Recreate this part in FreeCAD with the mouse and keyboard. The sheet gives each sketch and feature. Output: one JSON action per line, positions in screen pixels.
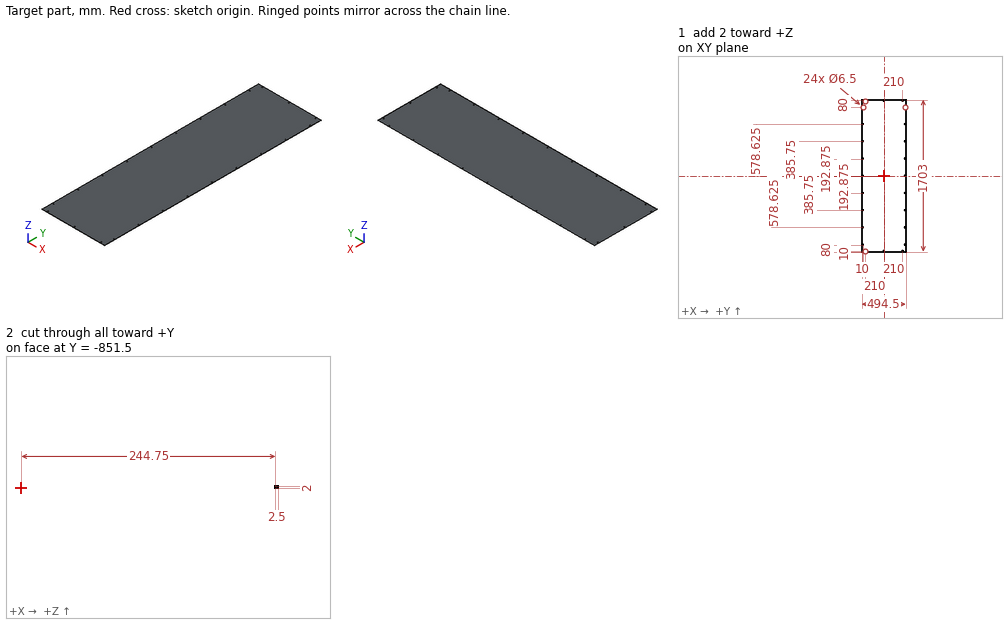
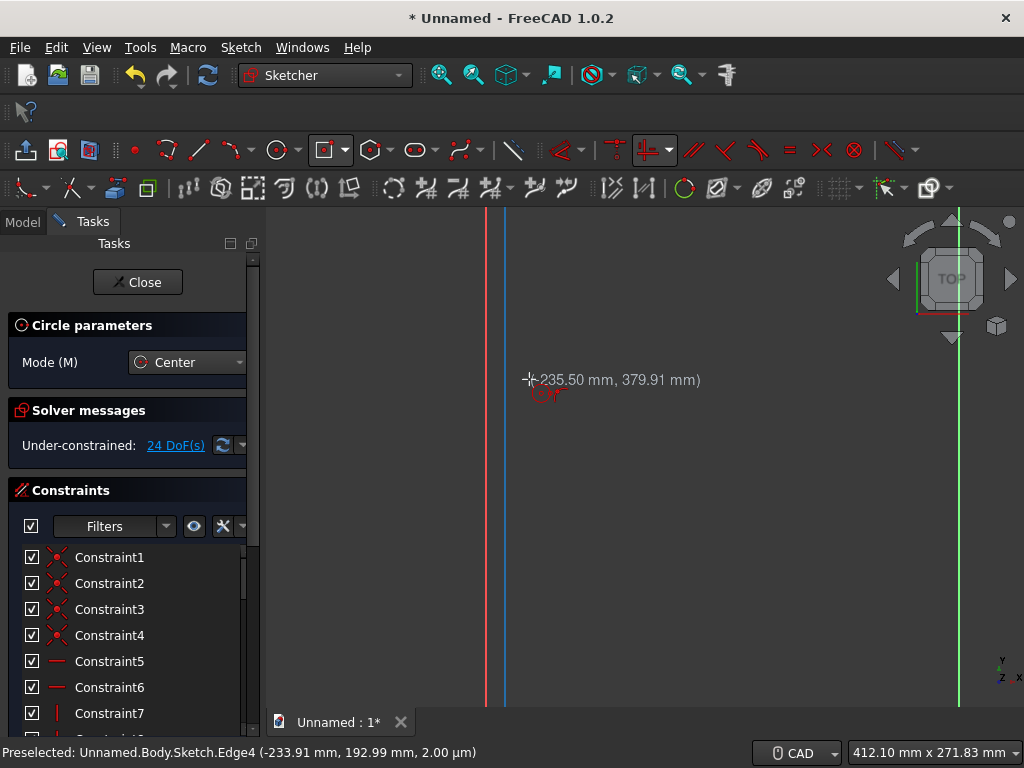
{"action": "left_click", "coordinate": [523, 375]}
{"action": "mouse_move", "coordinate": [527, 370]}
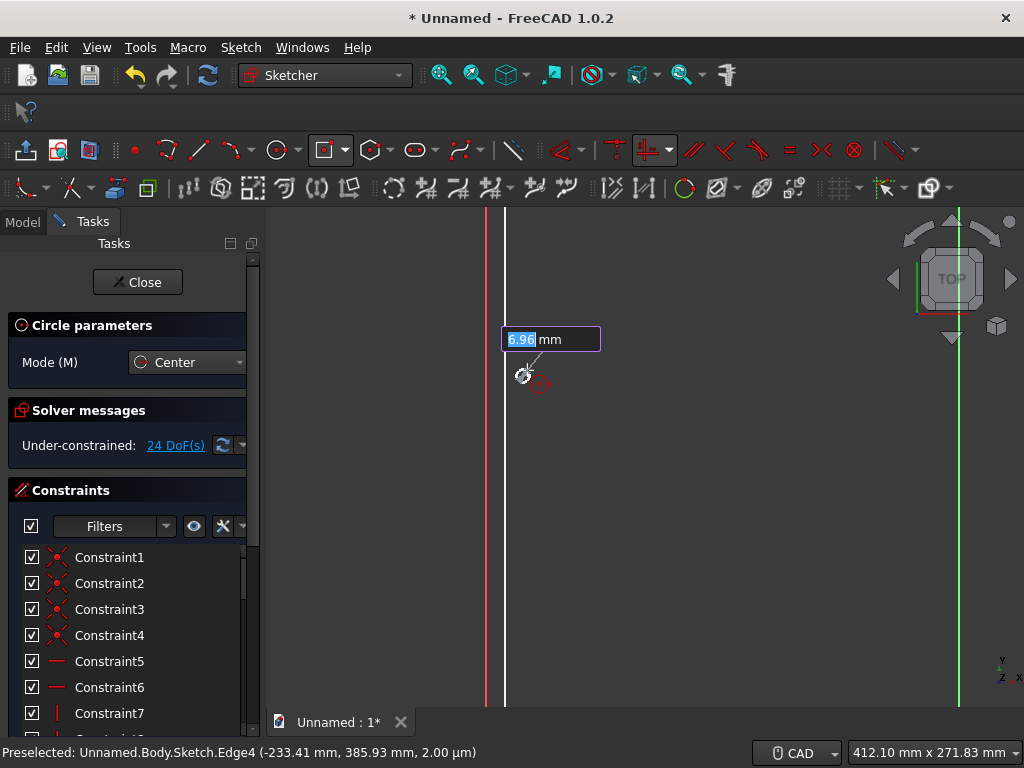
{"action": "type", "text": "6.5"}
{"action": "key", "text": "Return"}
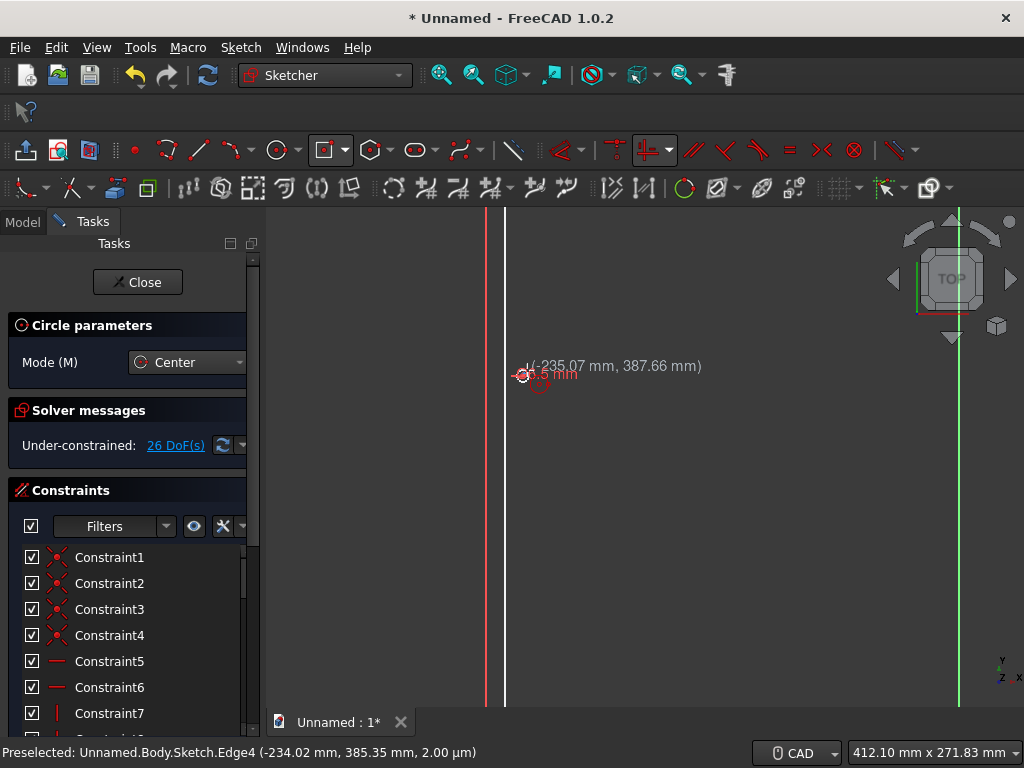
{"action": "scroll", "coordinate": [538, 394], "scroll_direction": "down", "scroll_amount": 12}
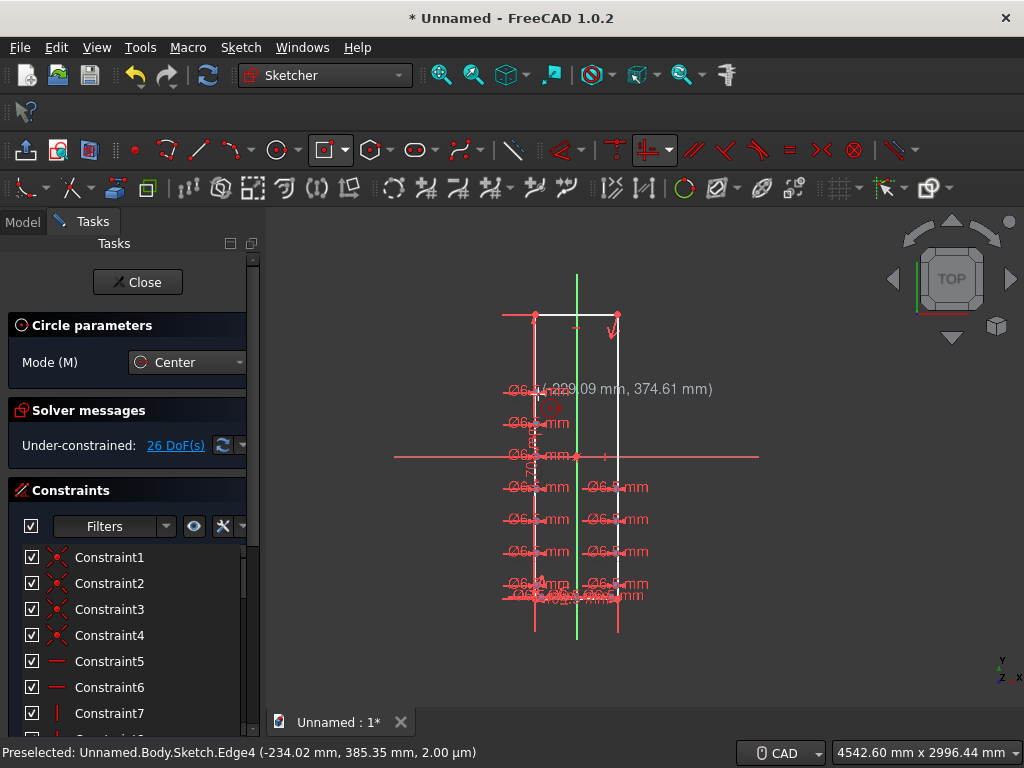
{"action": "scroll", "coordinate": [537, 360], "scroll_direction": "up", "scroll_amount": 19}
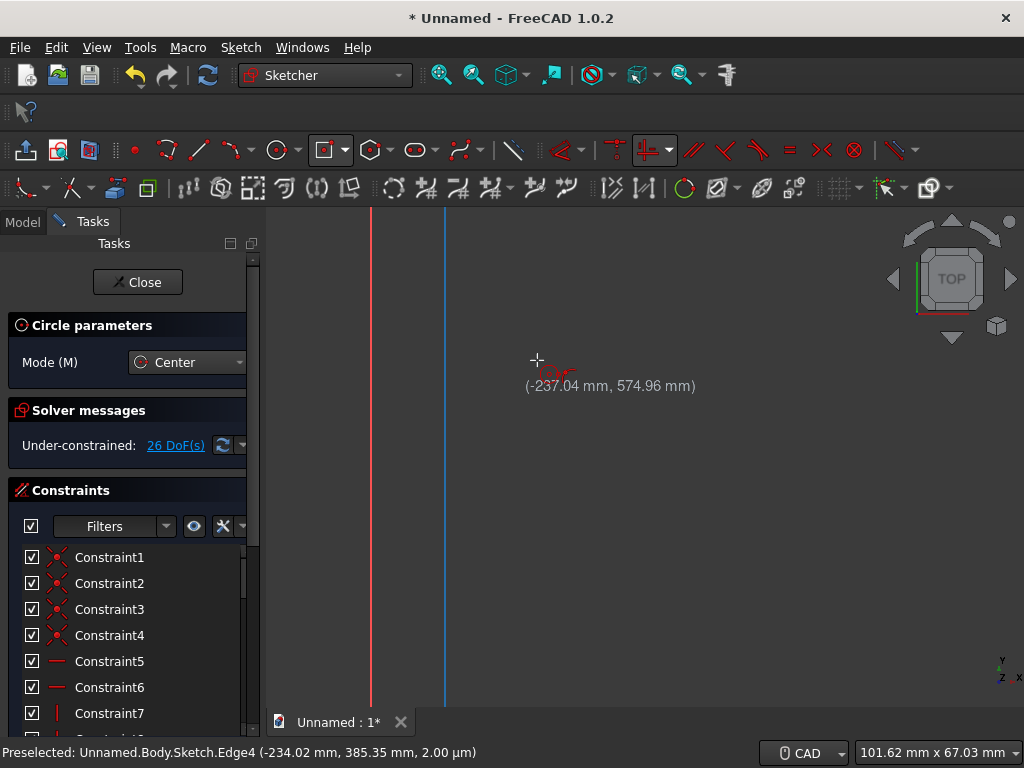
{"action": "scroll", "coordinate": [528, 338], "scroll_direction": "down", "scroll_amount": 18}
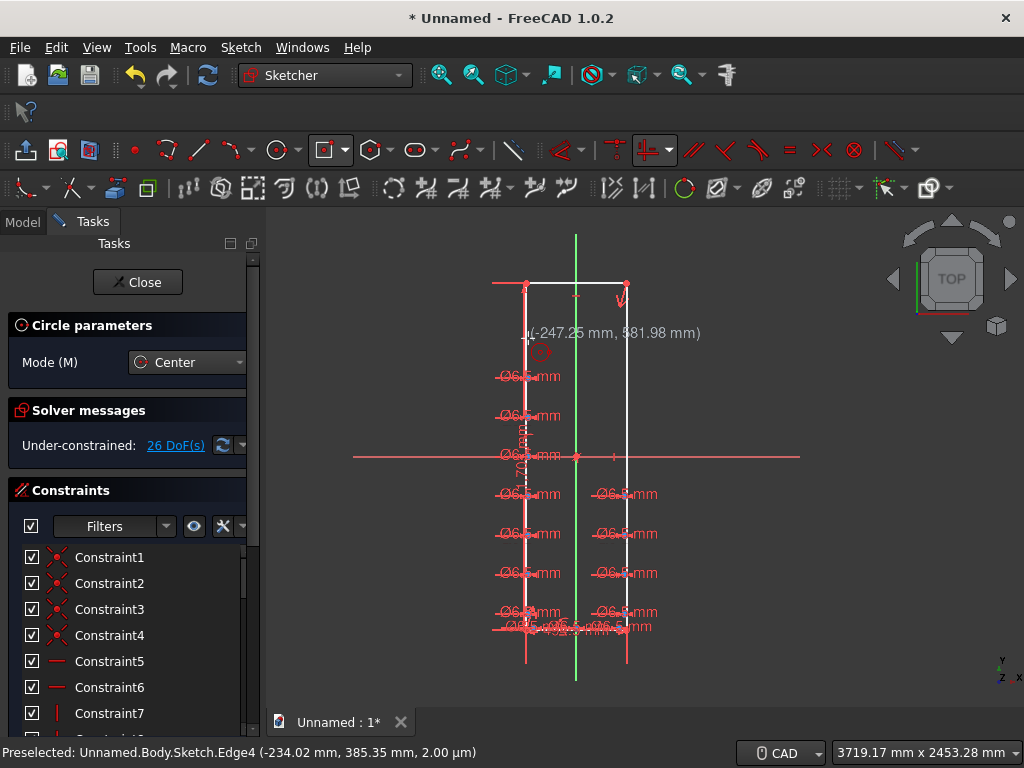
{"action": "scroll", "coordinate": [528, 339], "scroll_direction": "up", "scroll_amount": 11}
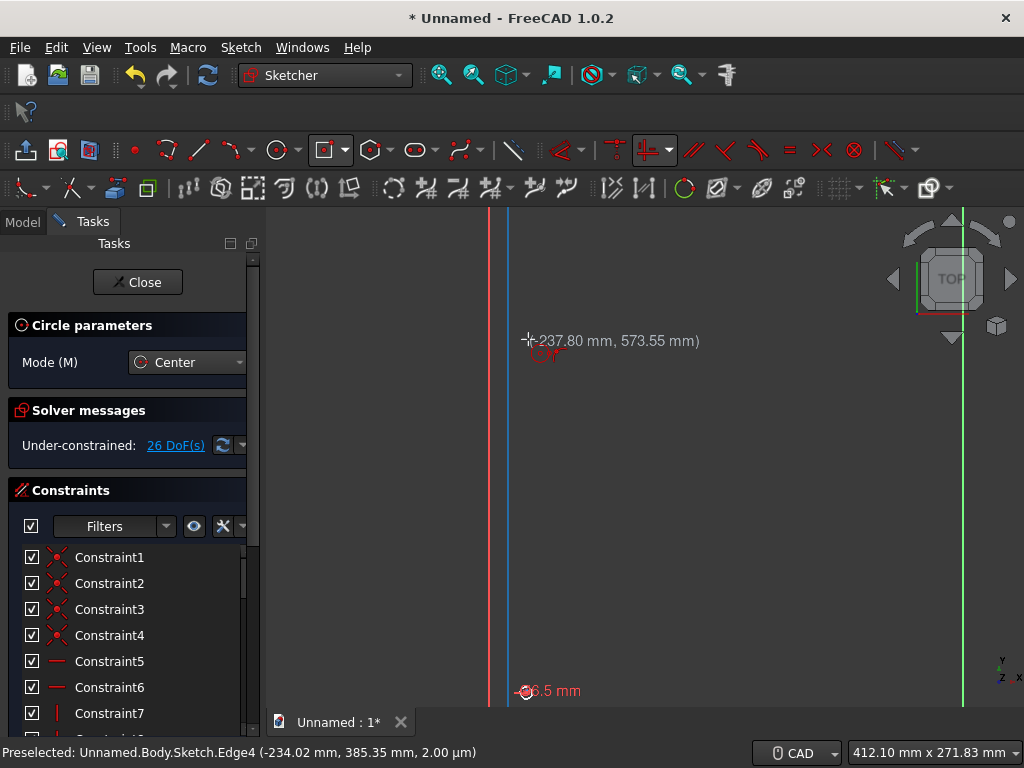
{"action": "left_click", "coordinate": [526, 337]}
{"action": "mouse_move", "coordinate": [530, 332]}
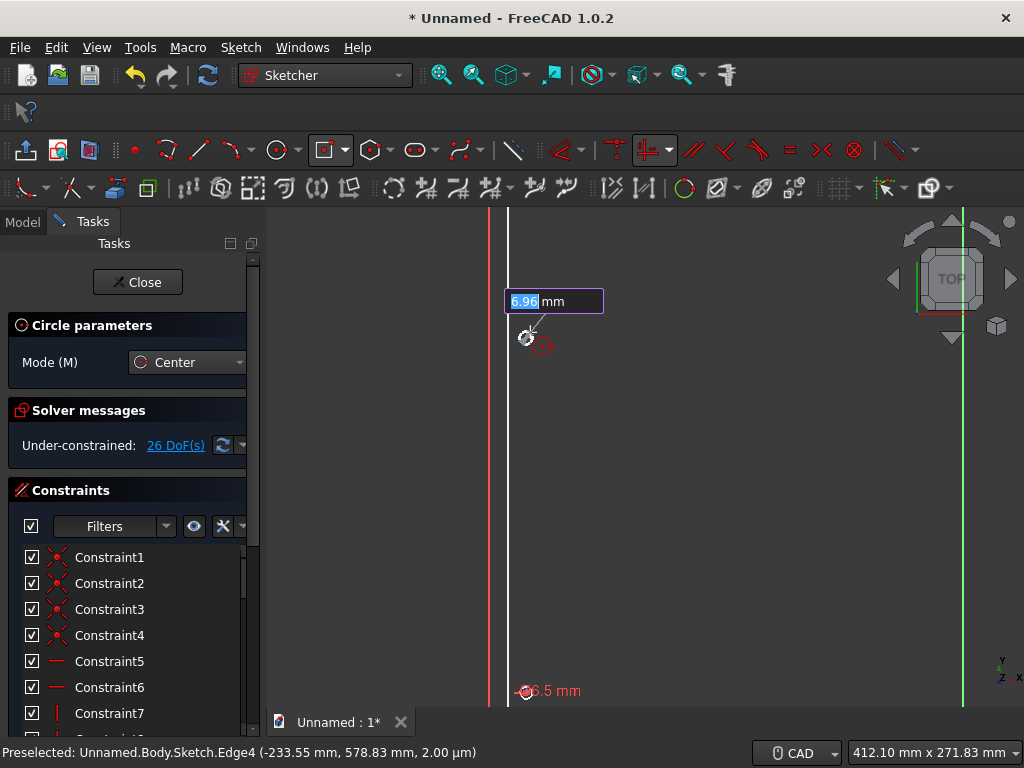
{"action": "type", "text": "6.5"}
{"action": "key", "text": "Return"}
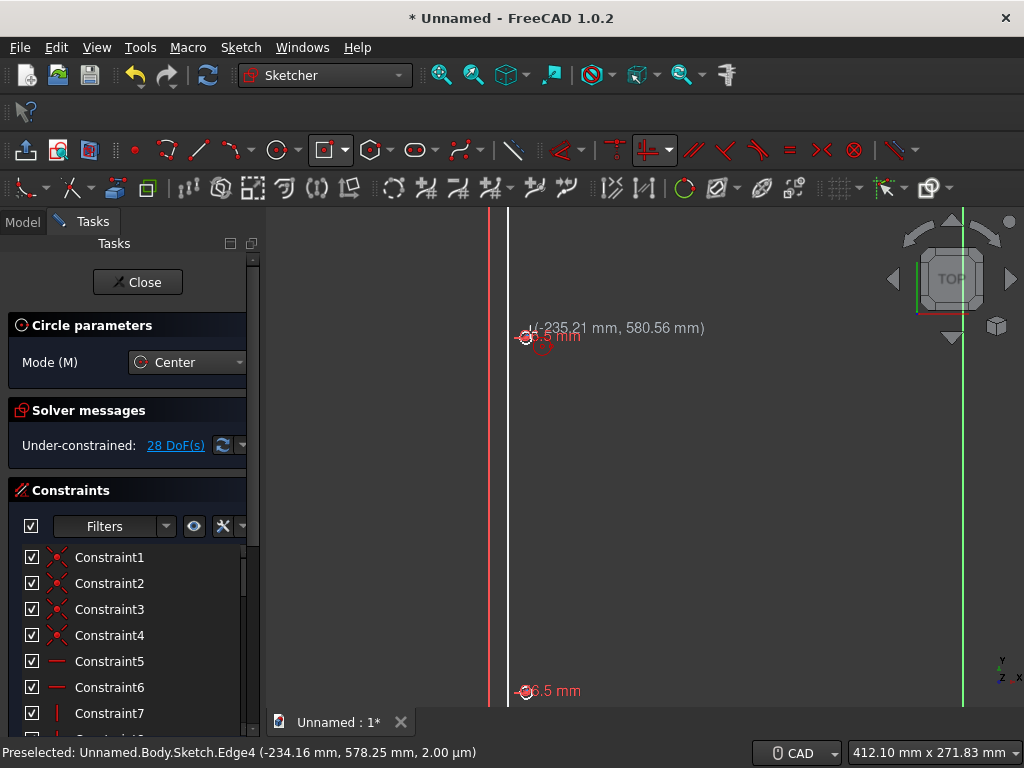
{"action": "scroll", "coordinate": [538, 363], "scroll_direction": "down", "scroll_amount": 12}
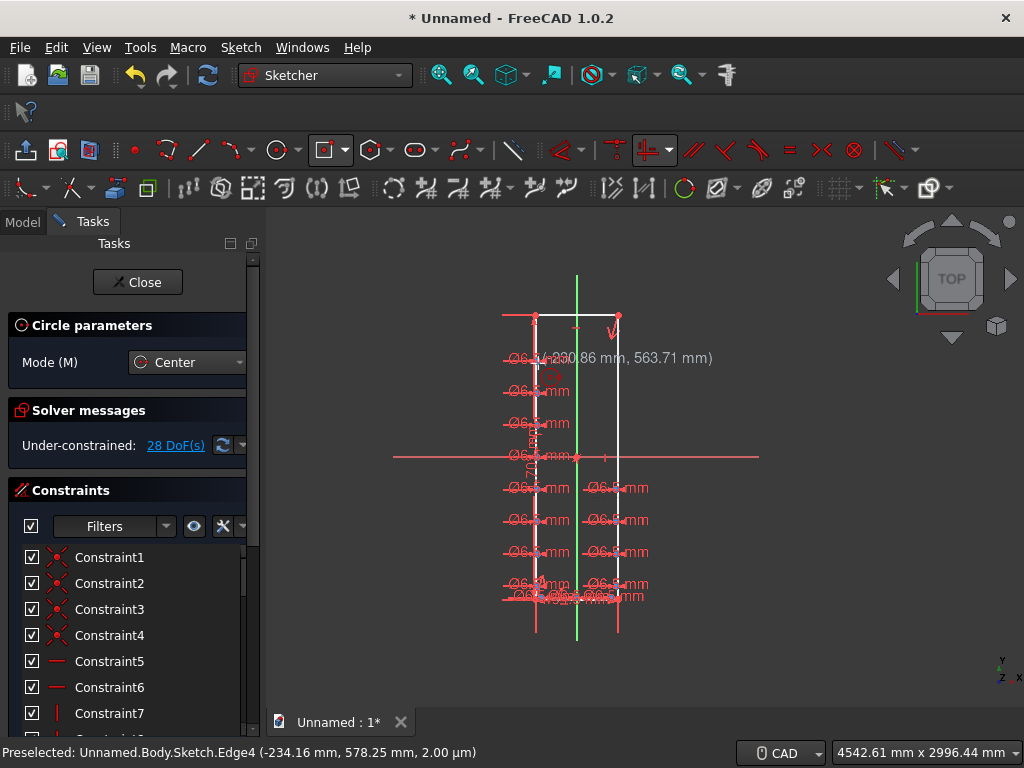
{"action": "scroll", "coordinate": [537, 329], "scroll_direction": "up", "scroll_amount": 19}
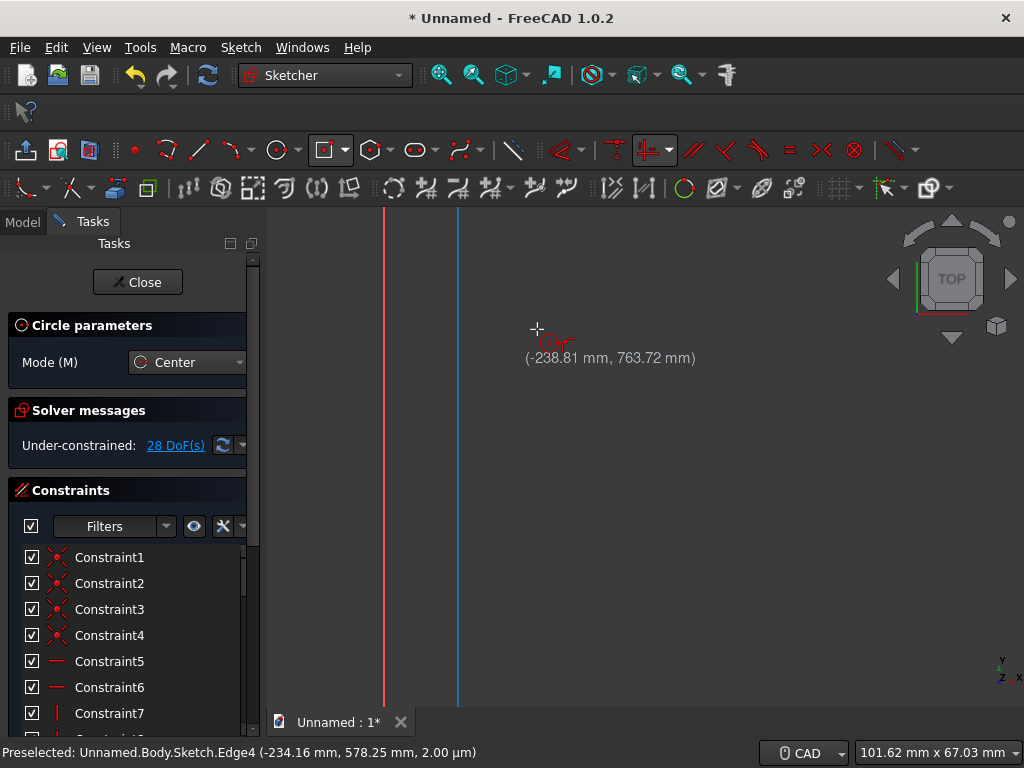
{"action": "scroll", "coordinate": [528, 300], "scroll_direction": "down", "scroll_amount": 18}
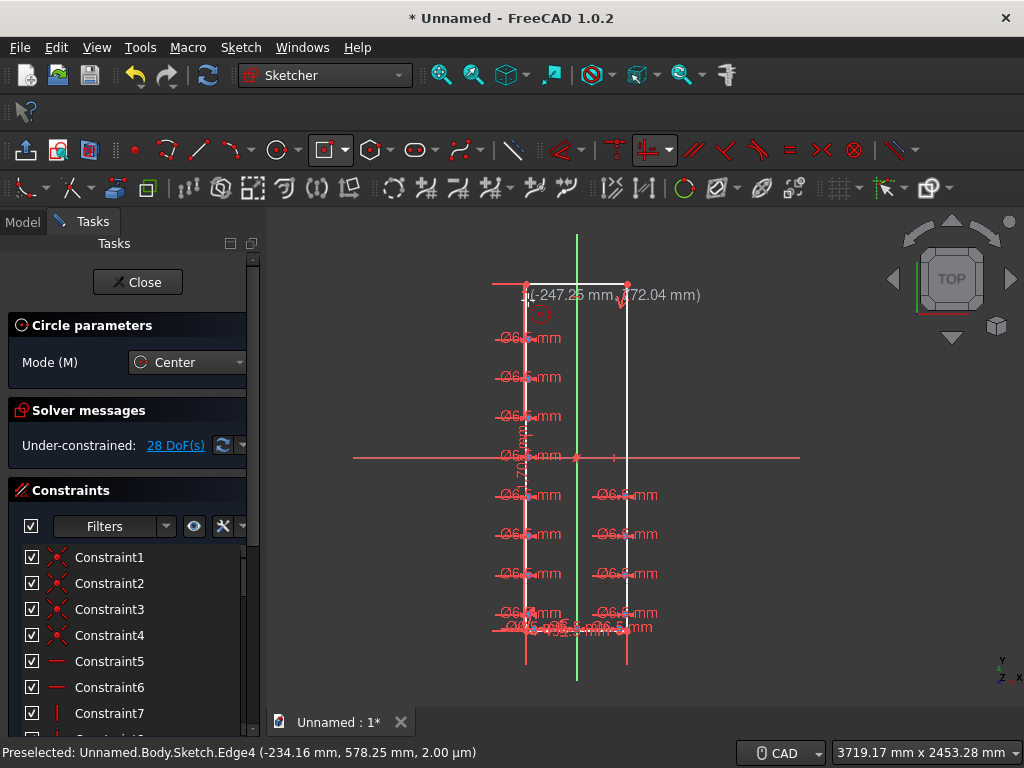
{"action": "scroll", "coordinate": [528, 300], "scroll_direction": "up", "scroll_amount": 11}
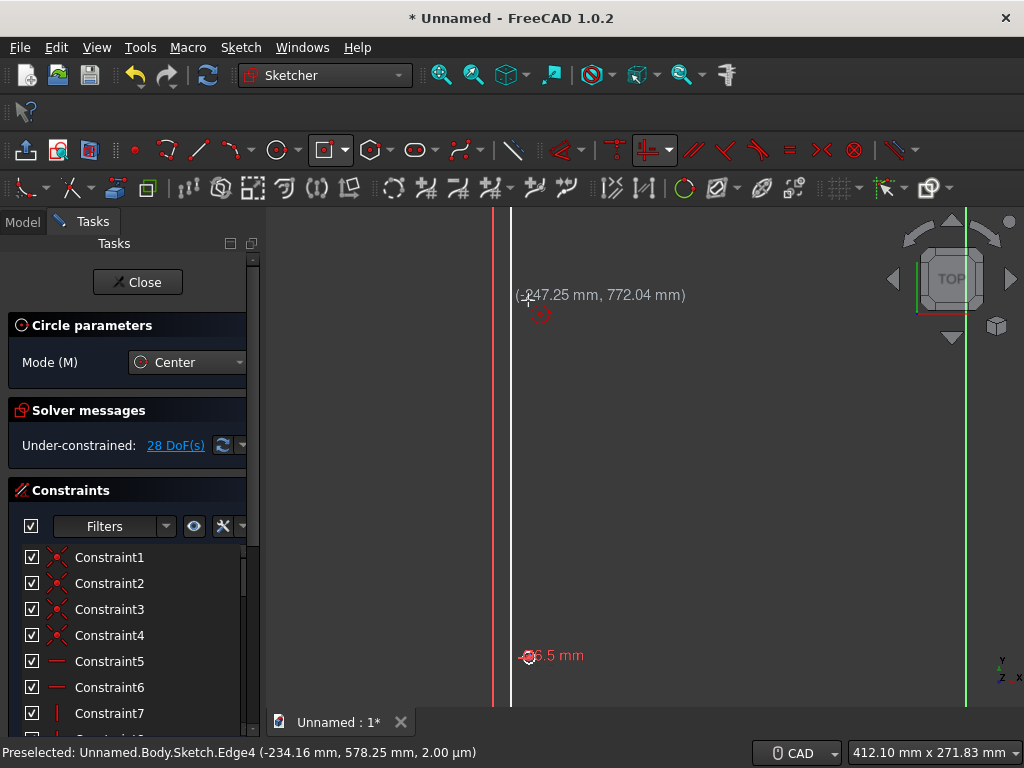
{"action": "left_click", "coordinate": [529, 301]}
{"action": "mouse_move", "coordinate": [534, 297]}